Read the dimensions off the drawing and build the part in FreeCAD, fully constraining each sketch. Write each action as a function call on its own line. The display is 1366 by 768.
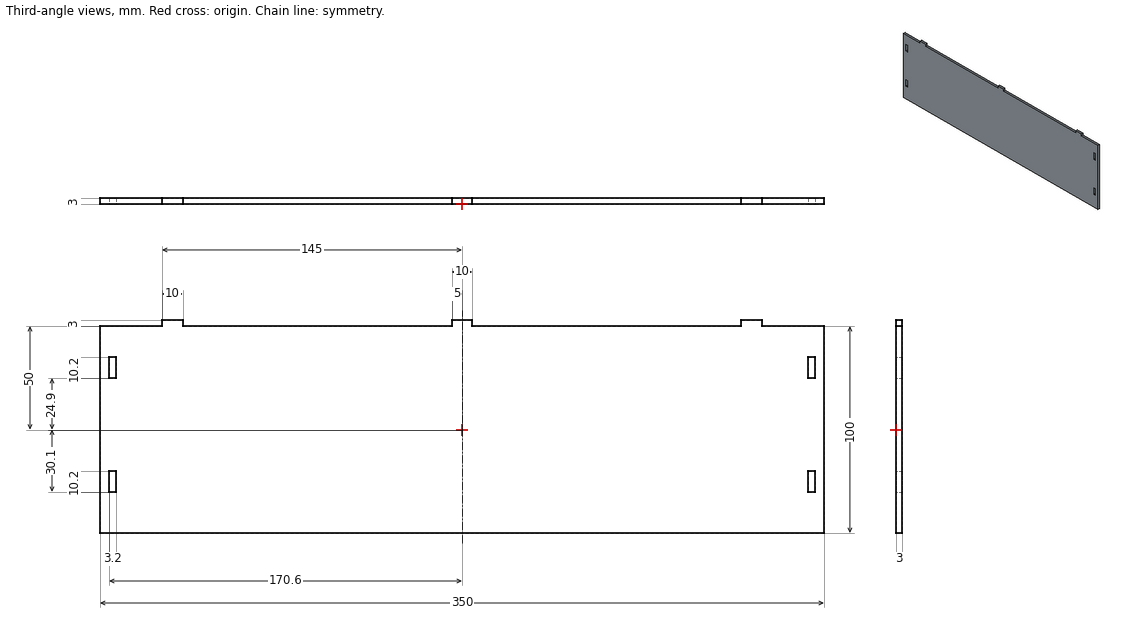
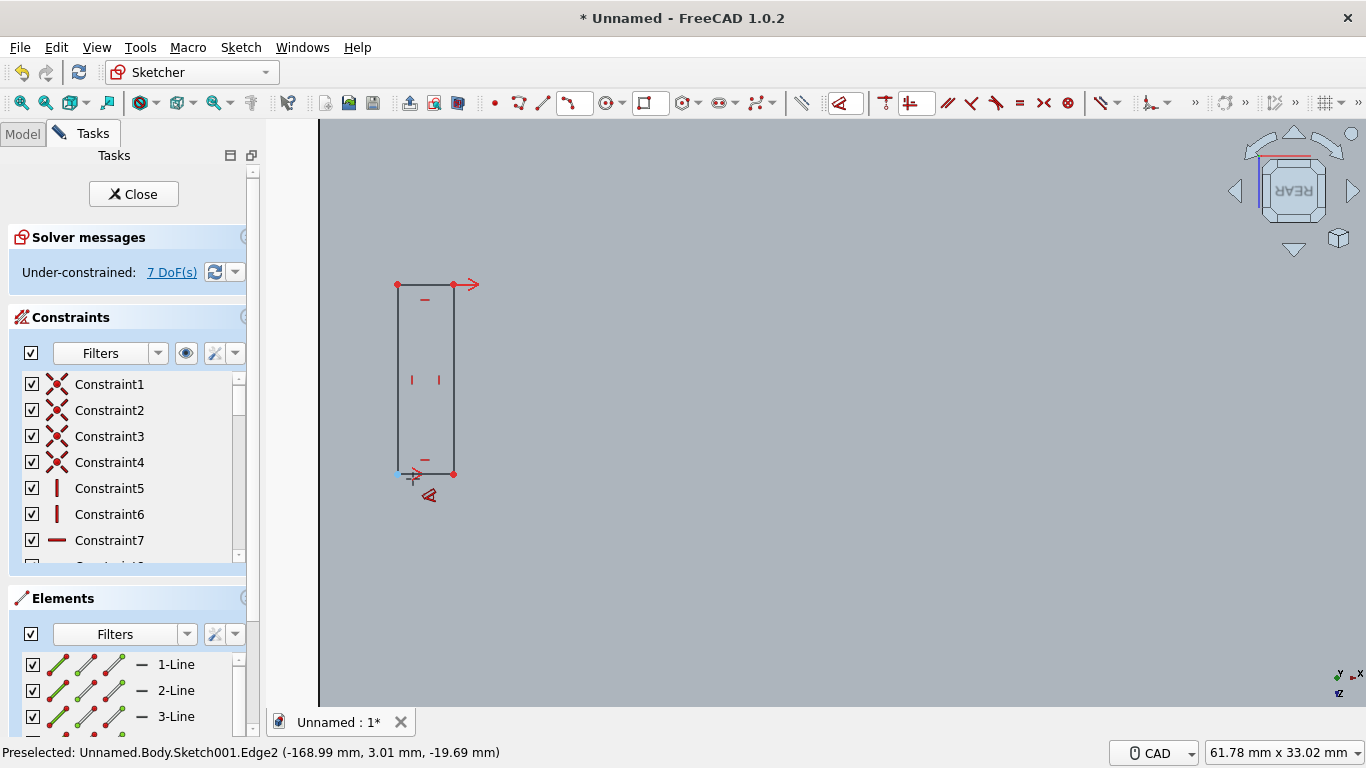
click(414, 474)
click(426, 508)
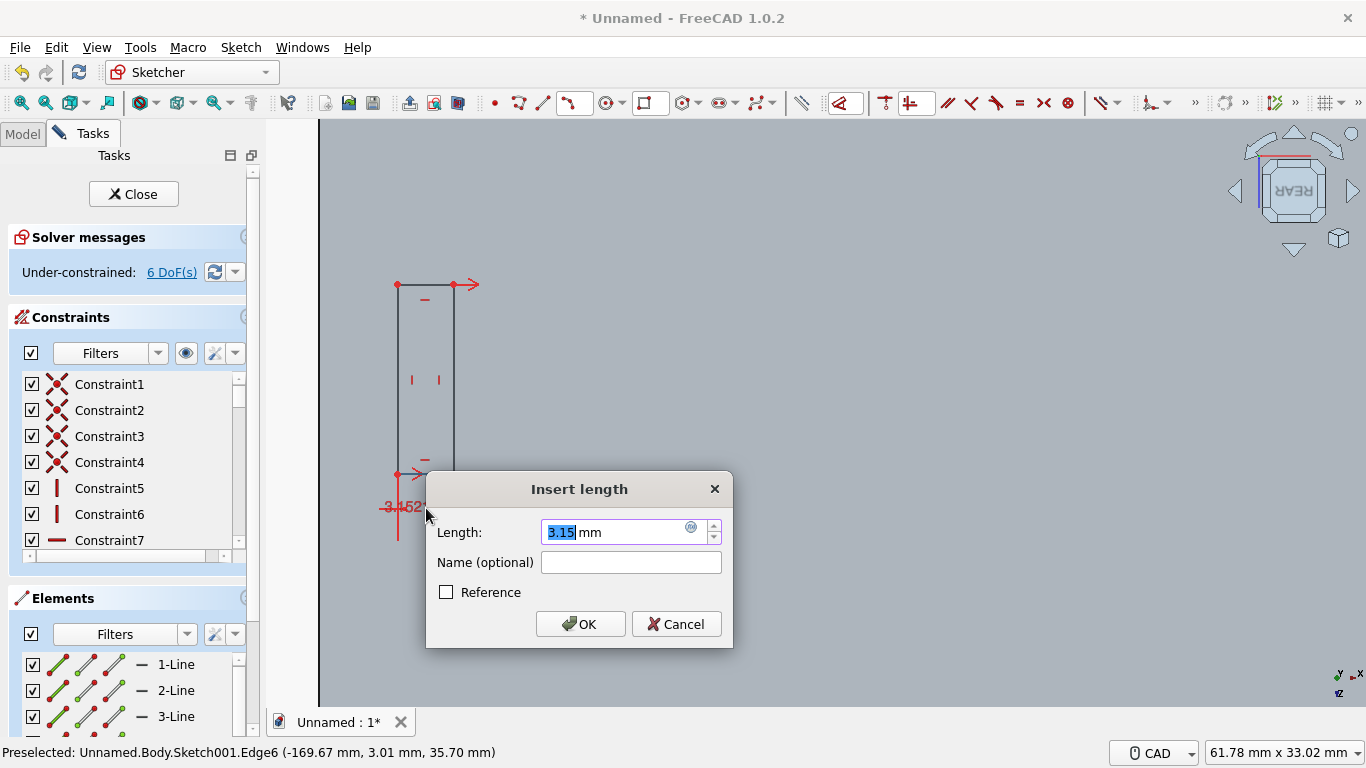
text(3.2)
key(Return)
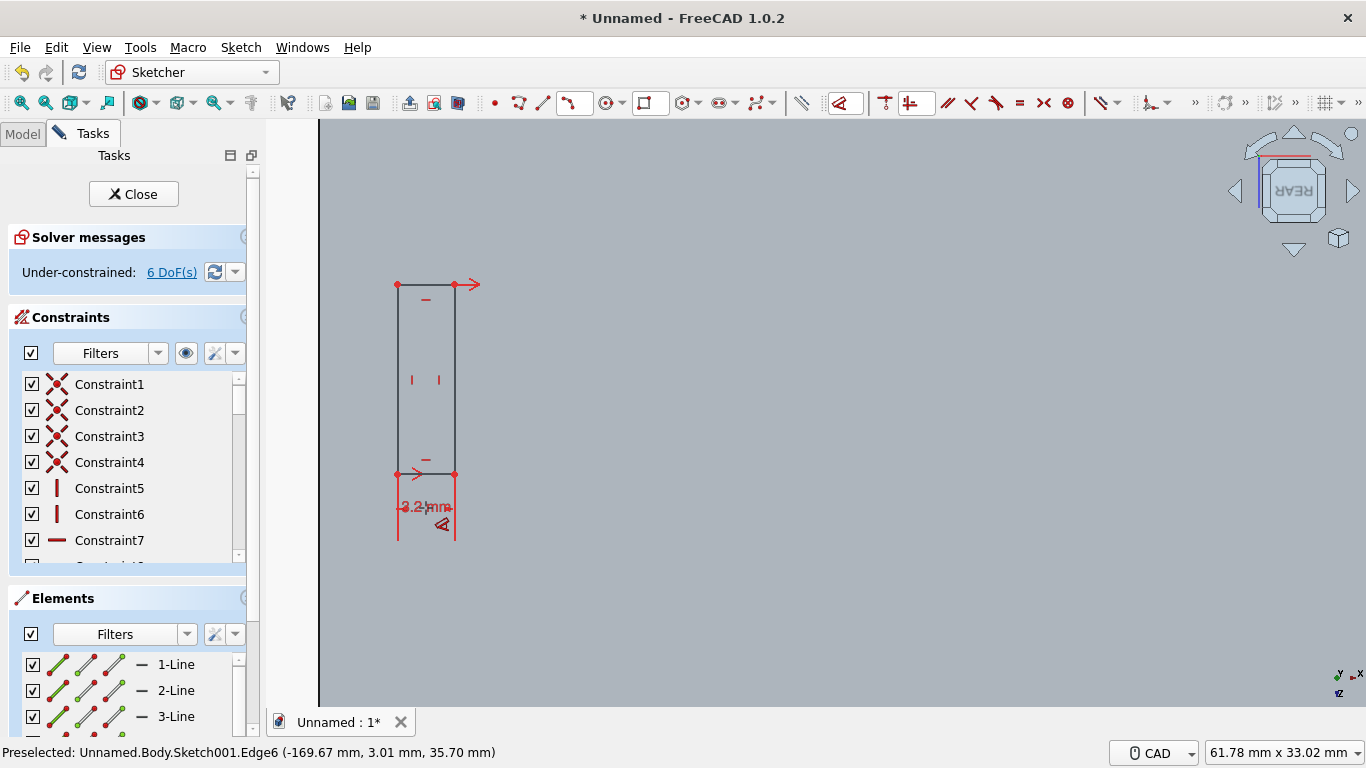
scroll(413, 479, down, 11)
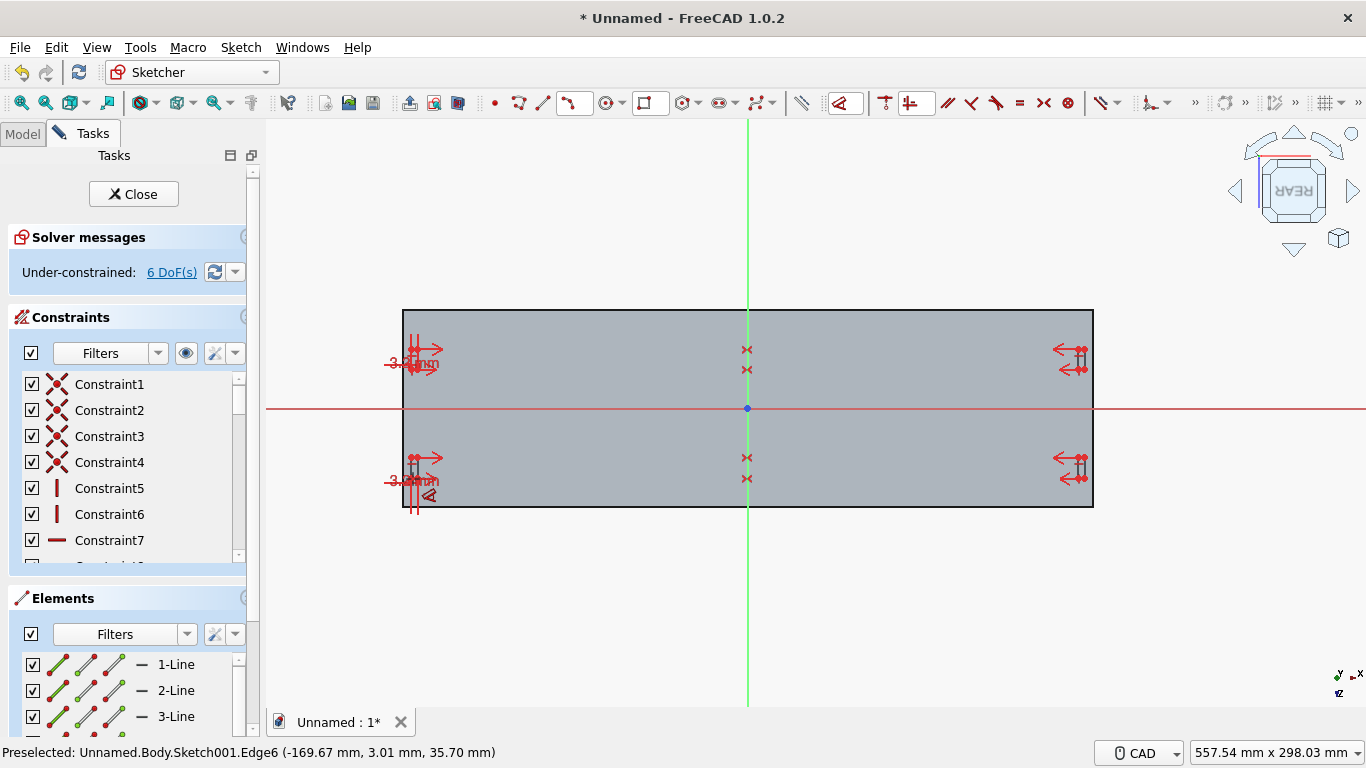
scroll(411, 356, up, 5)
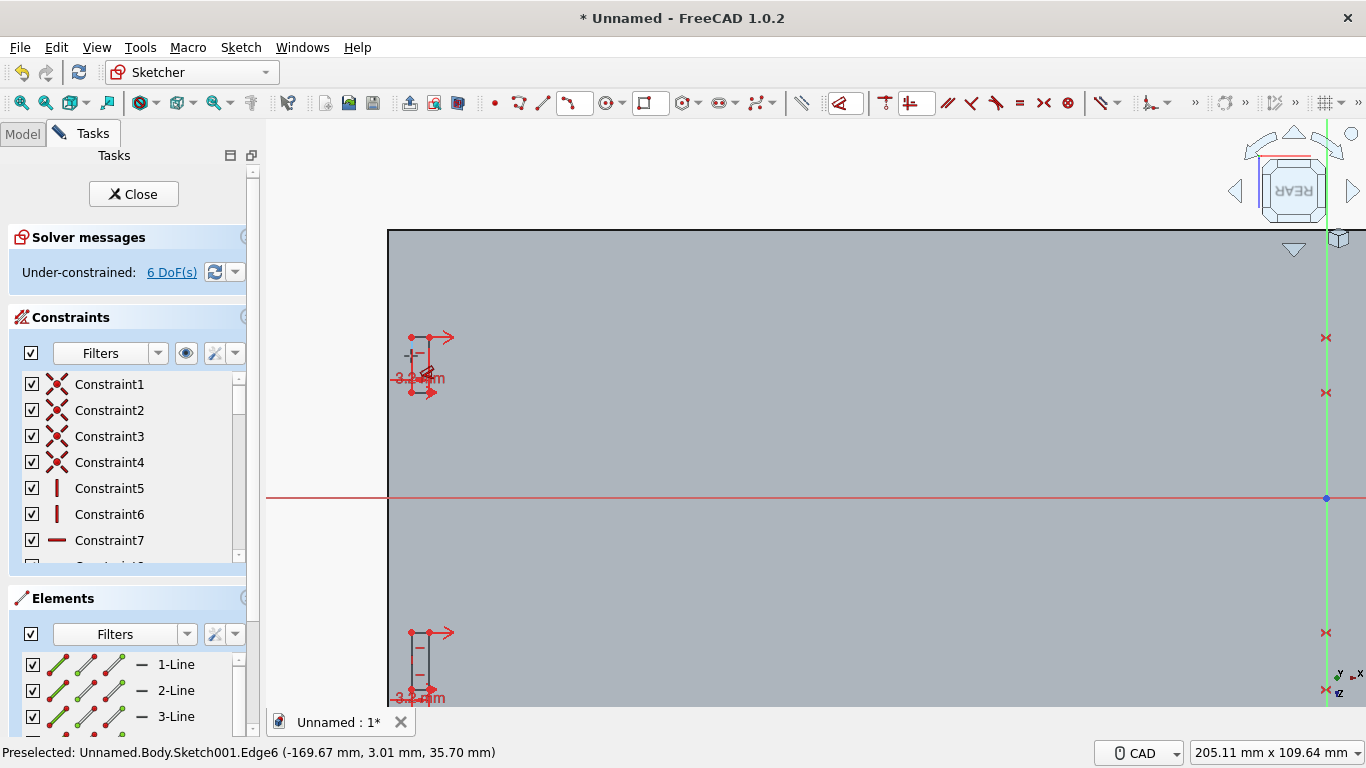
click(412, 354)
click(378, 352)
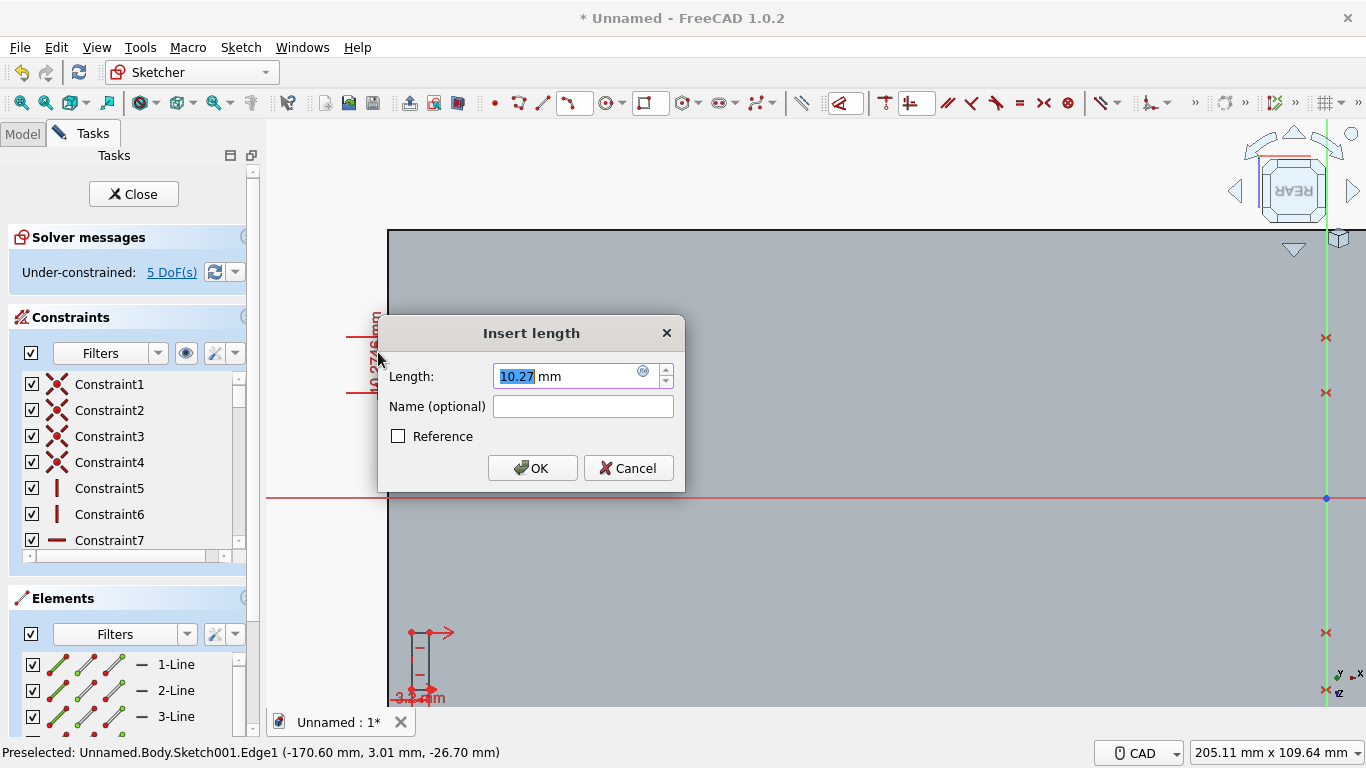
text(10.2)
key(Return)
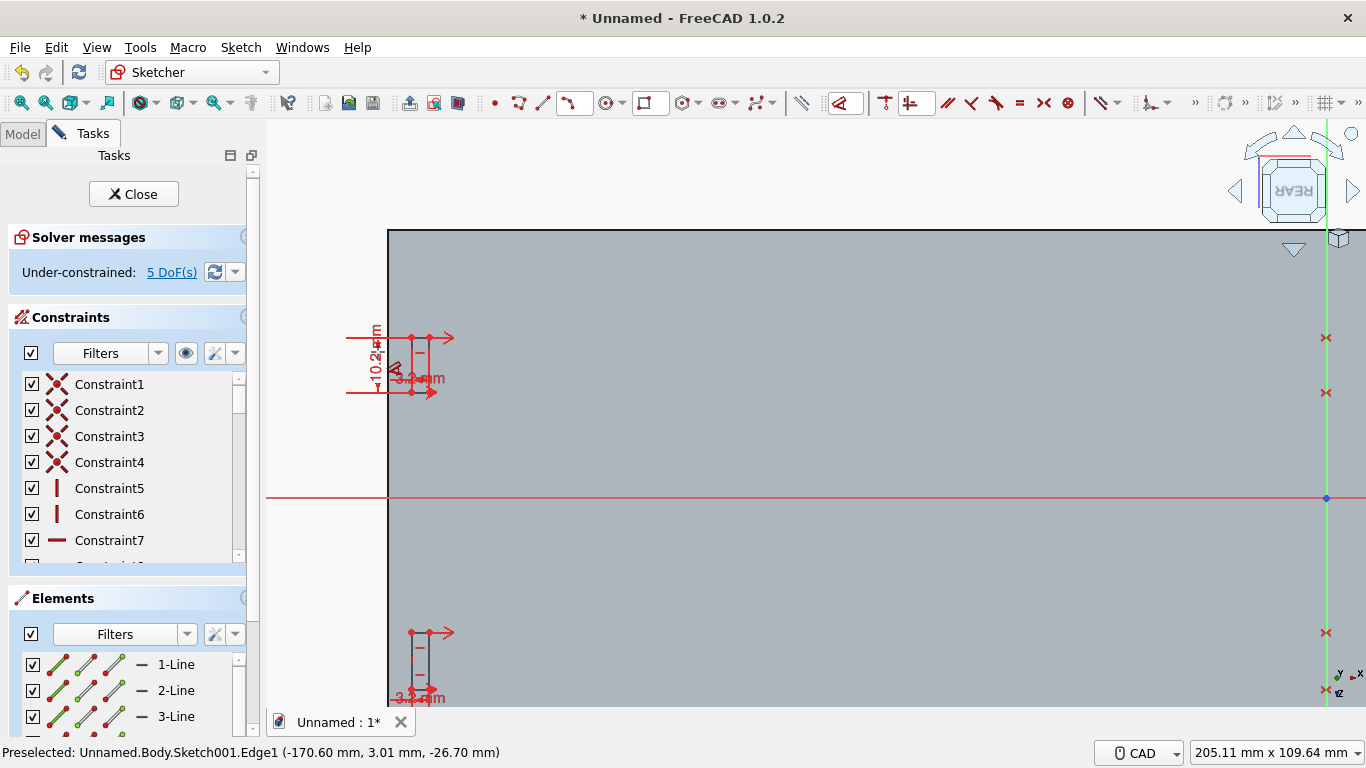
click(412, 650)
click(378, 656)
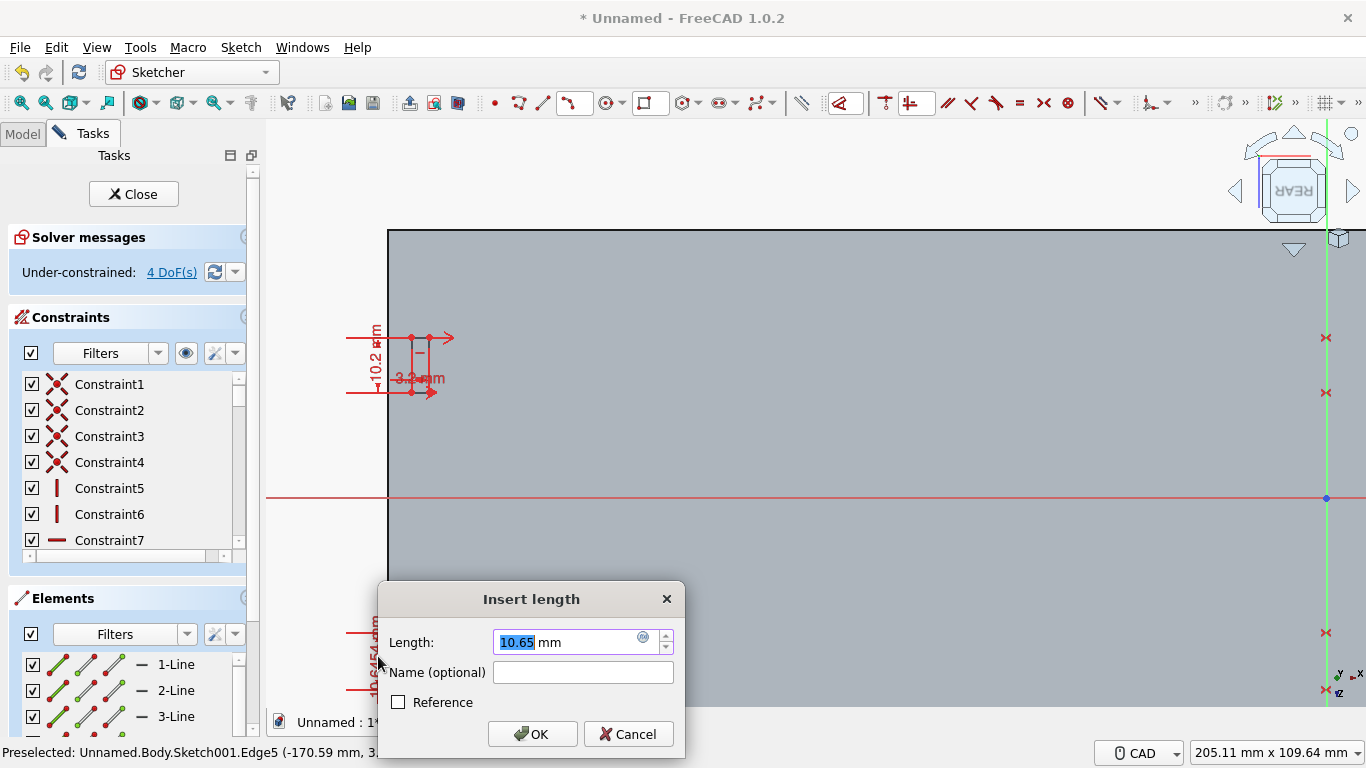
text(10.2)
key(Return)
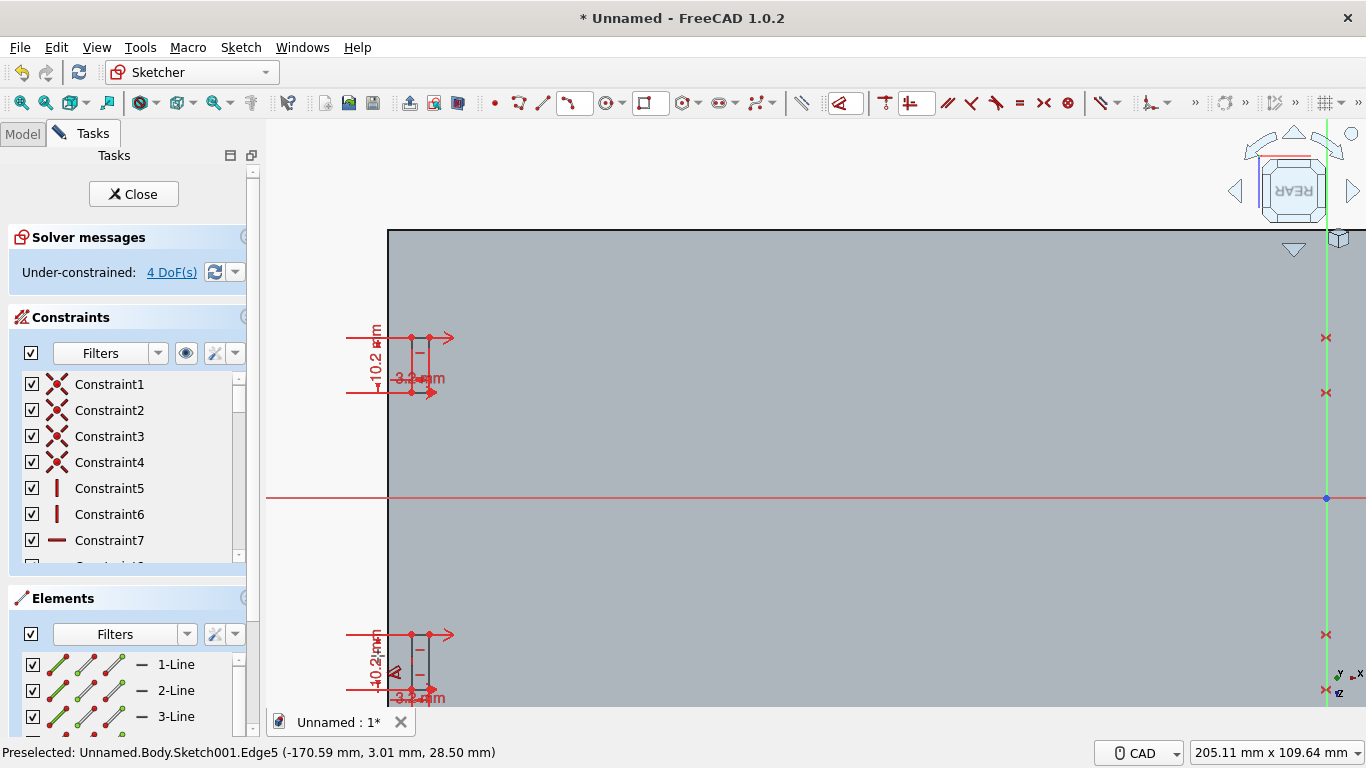
click(412, 338)
click(378, 418)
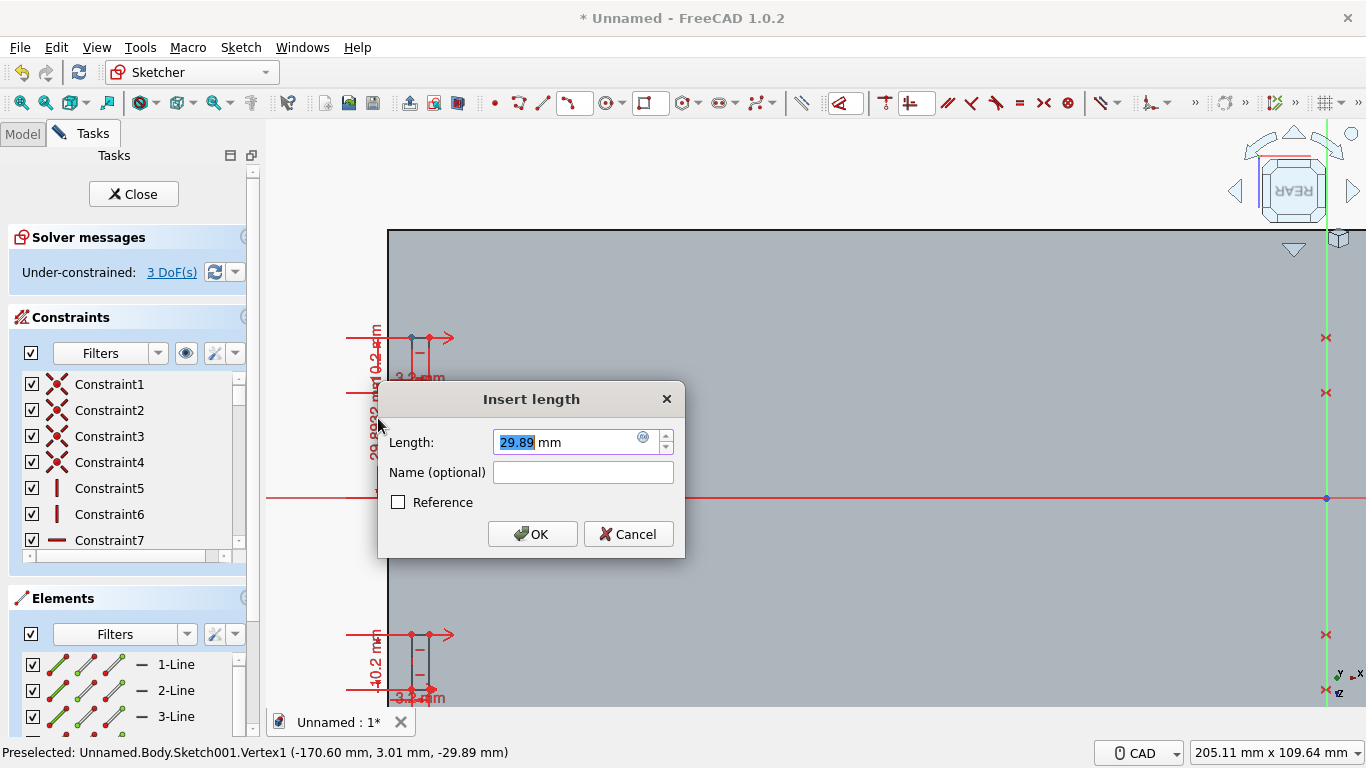
text(30.1)
key(Return)